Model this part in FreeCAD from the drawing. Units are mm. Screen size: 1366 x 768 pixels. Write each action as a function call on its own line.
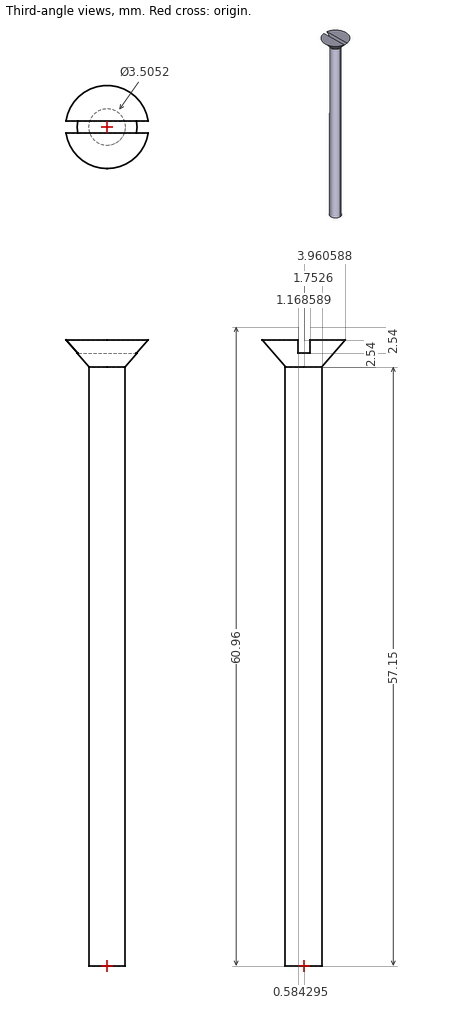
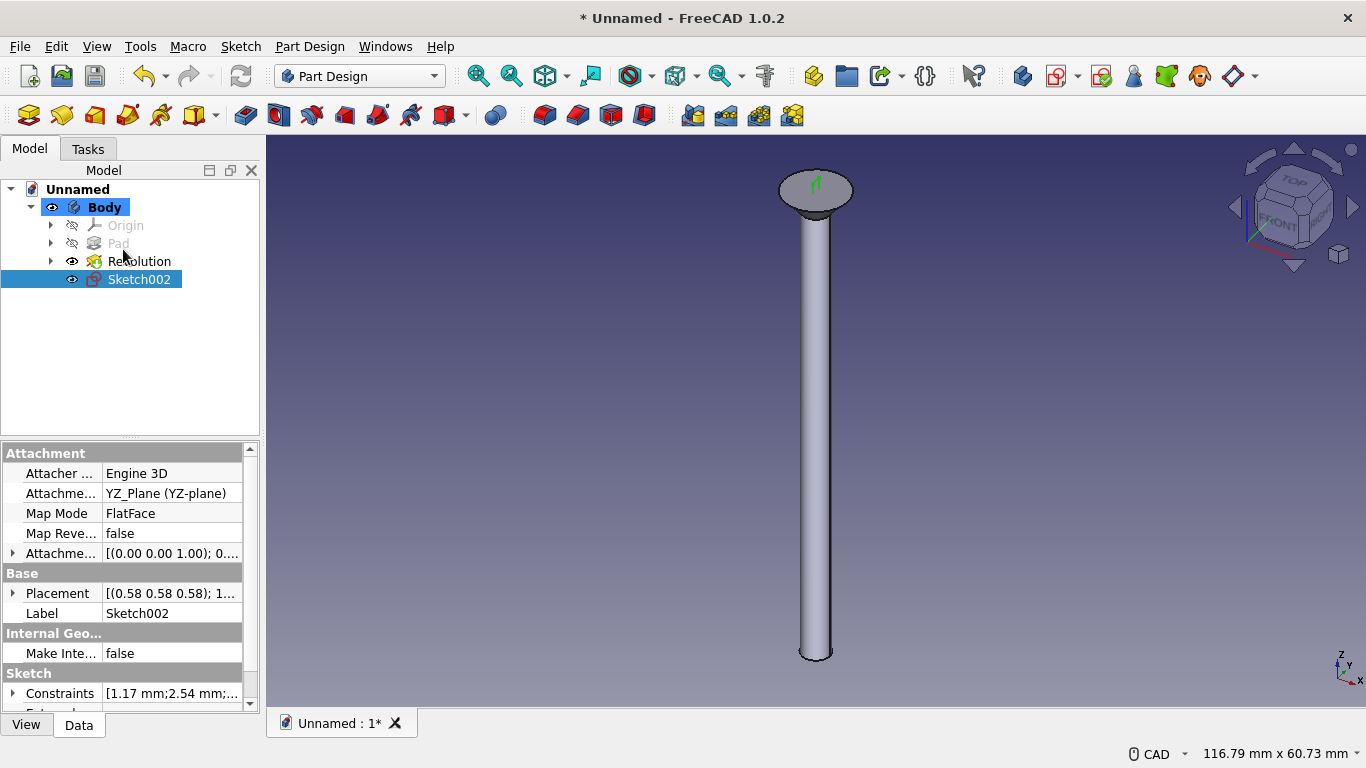
click(246, 116)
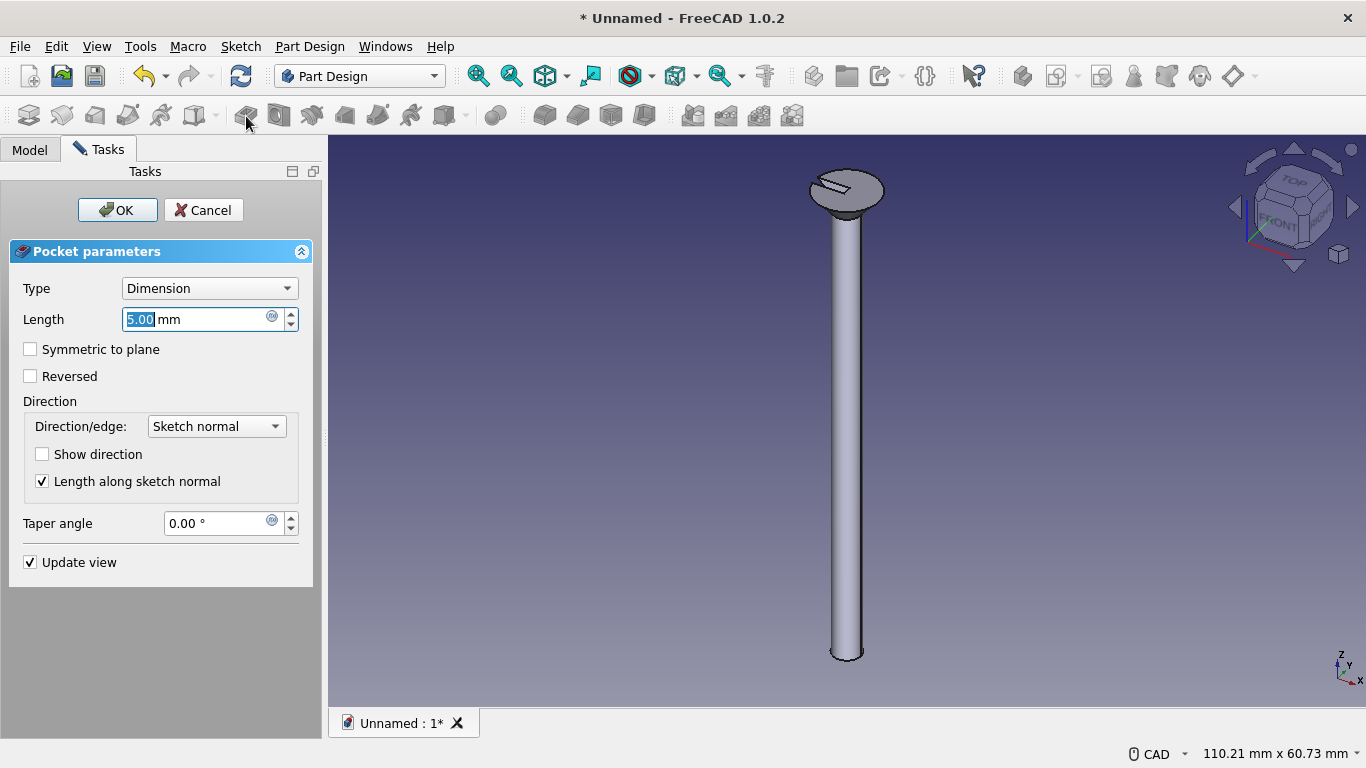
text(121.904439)
key(Tab)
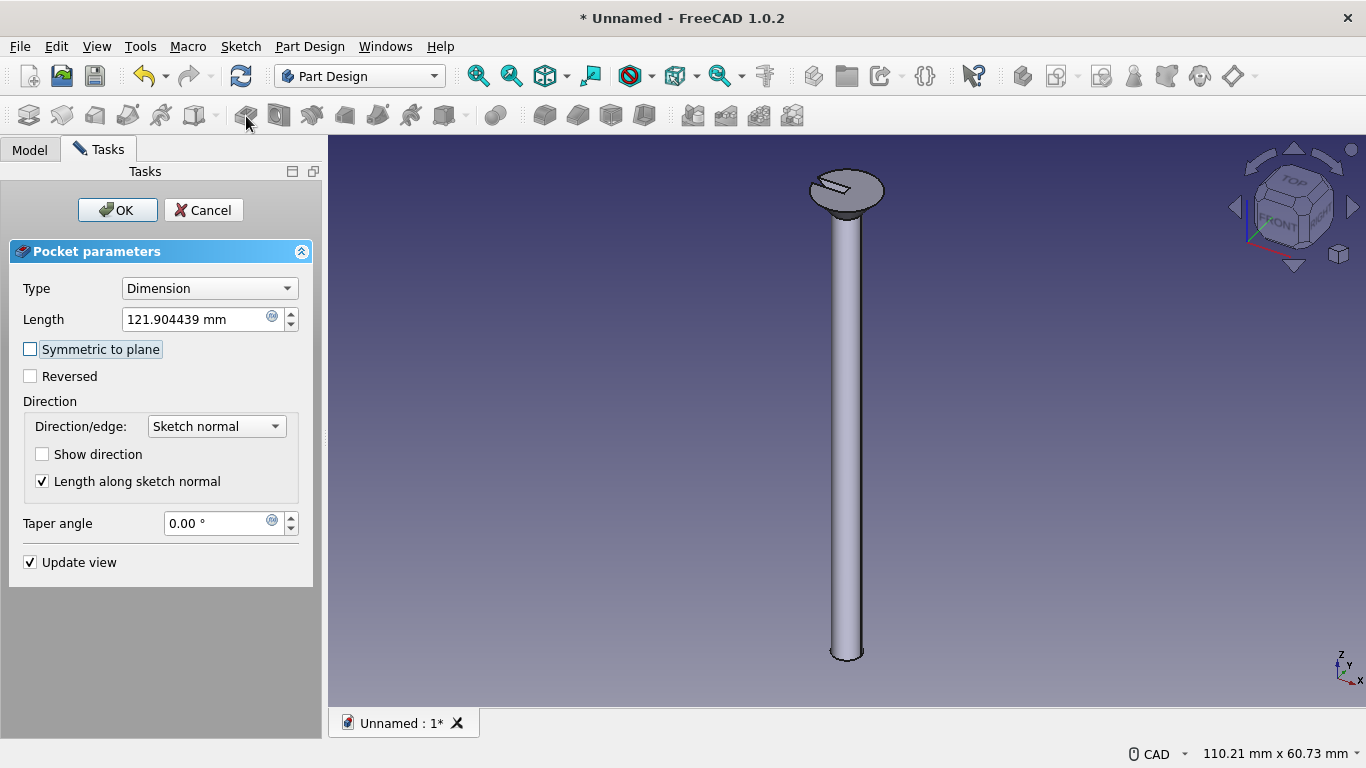
click(31, 349)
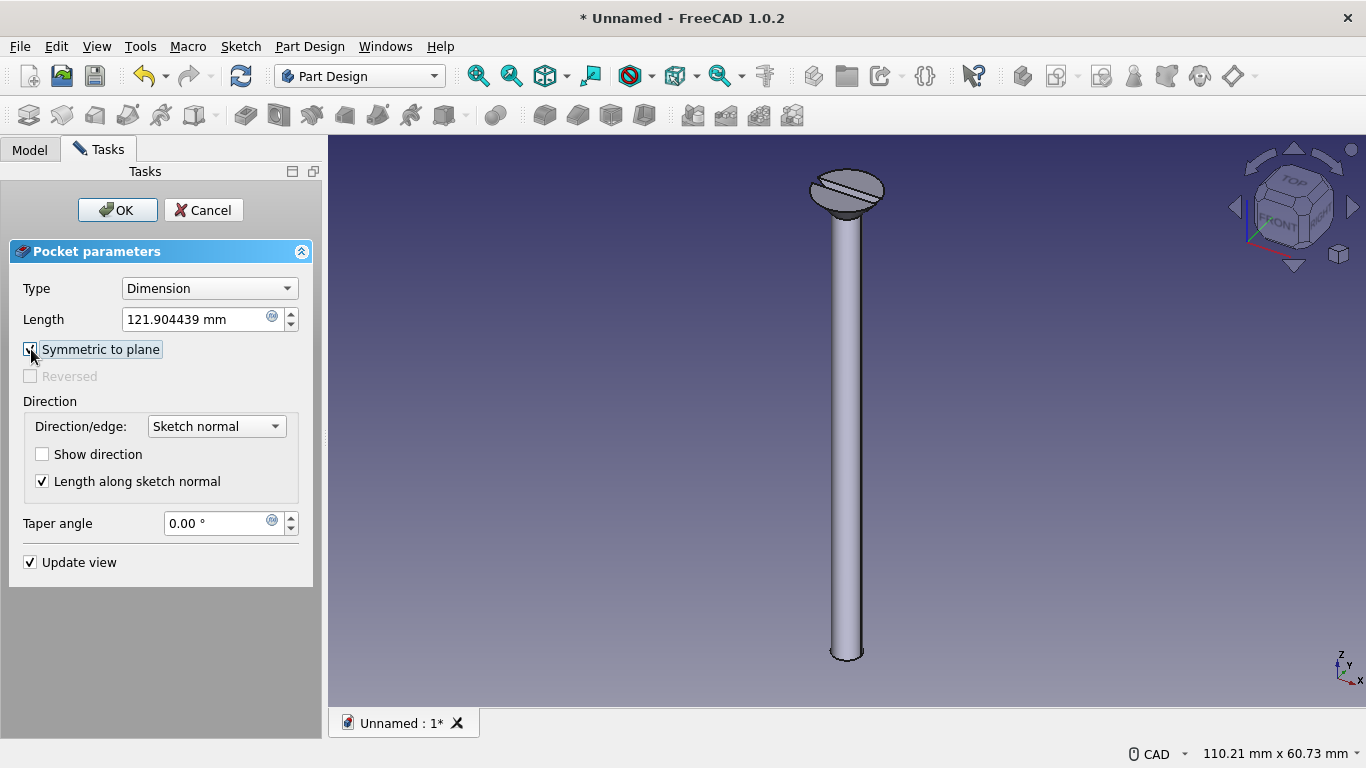
click(118, 210)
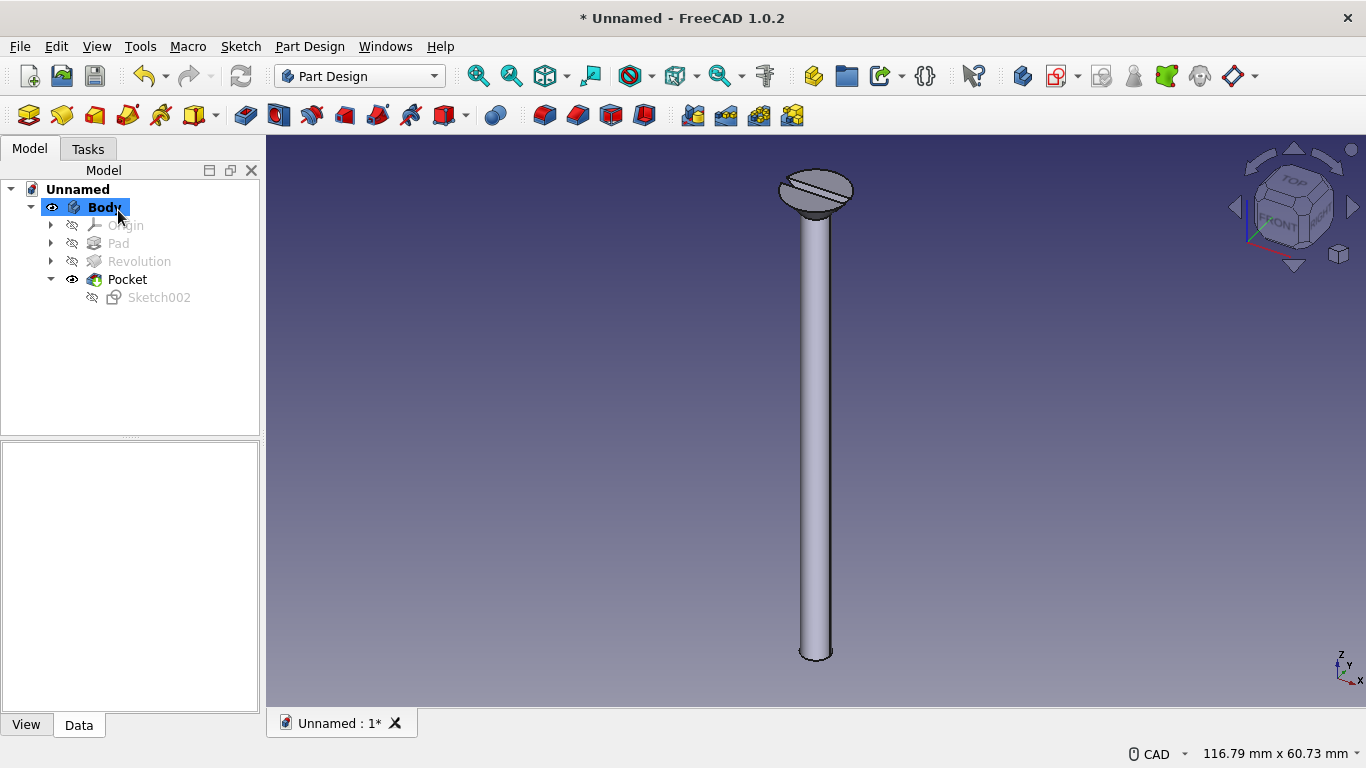
key(0)